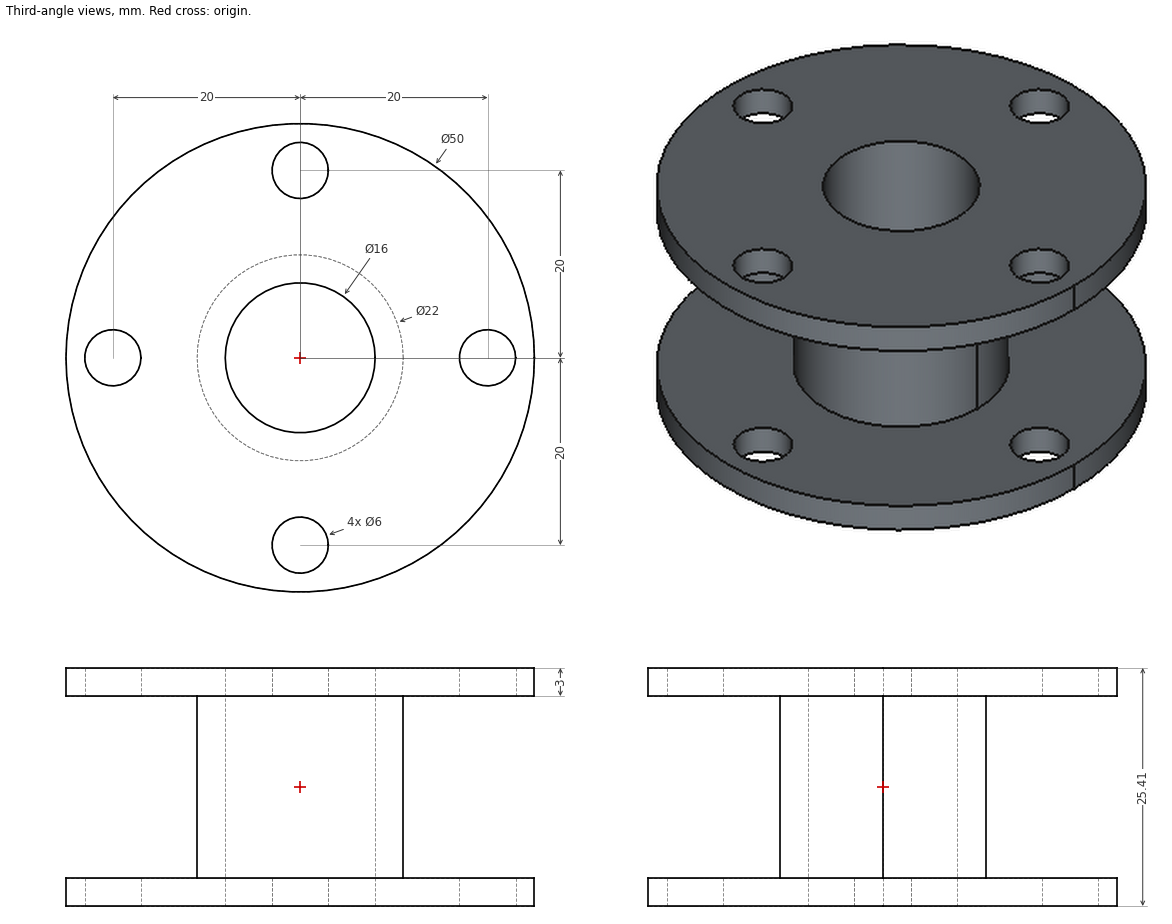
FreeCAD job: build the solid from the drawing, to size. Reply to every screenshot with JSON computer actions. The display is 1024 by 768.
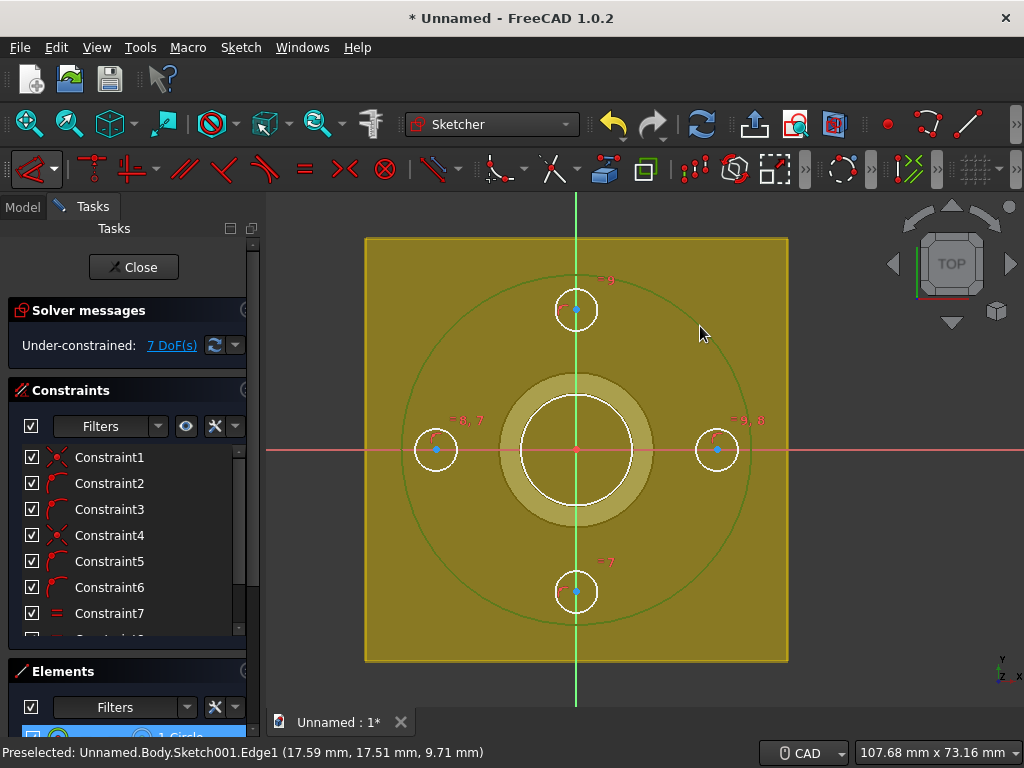
{"action": "left_click", "coordinate": [56, 170]}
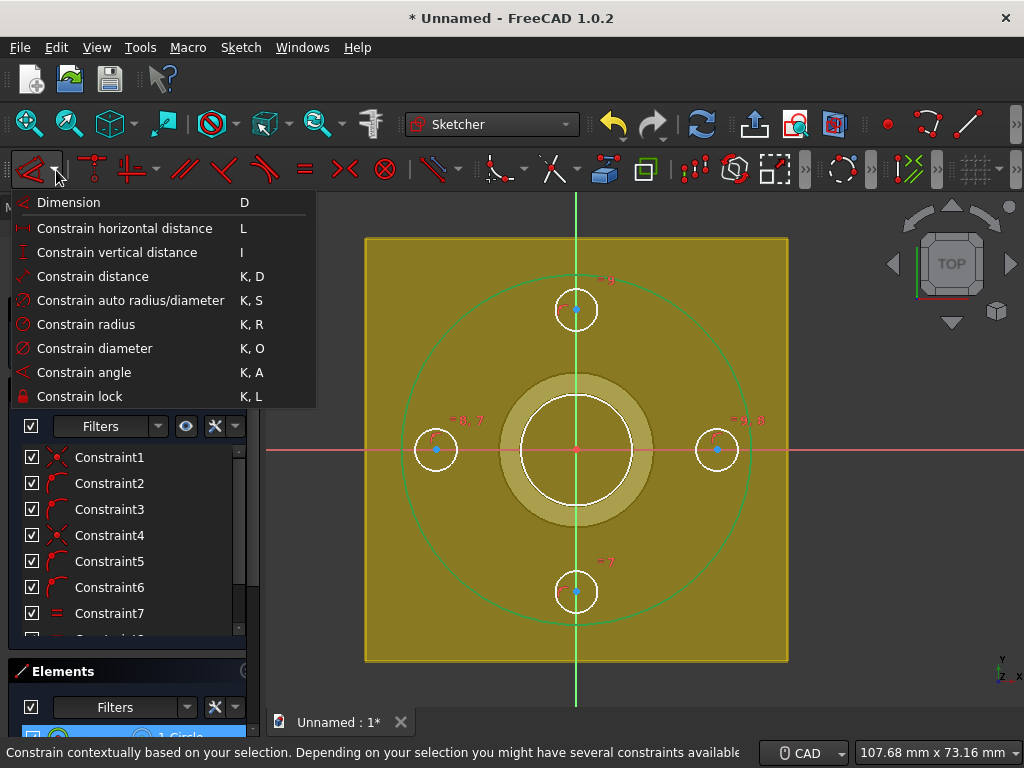
{"action": "left_click", "coordinate": [164, 348]}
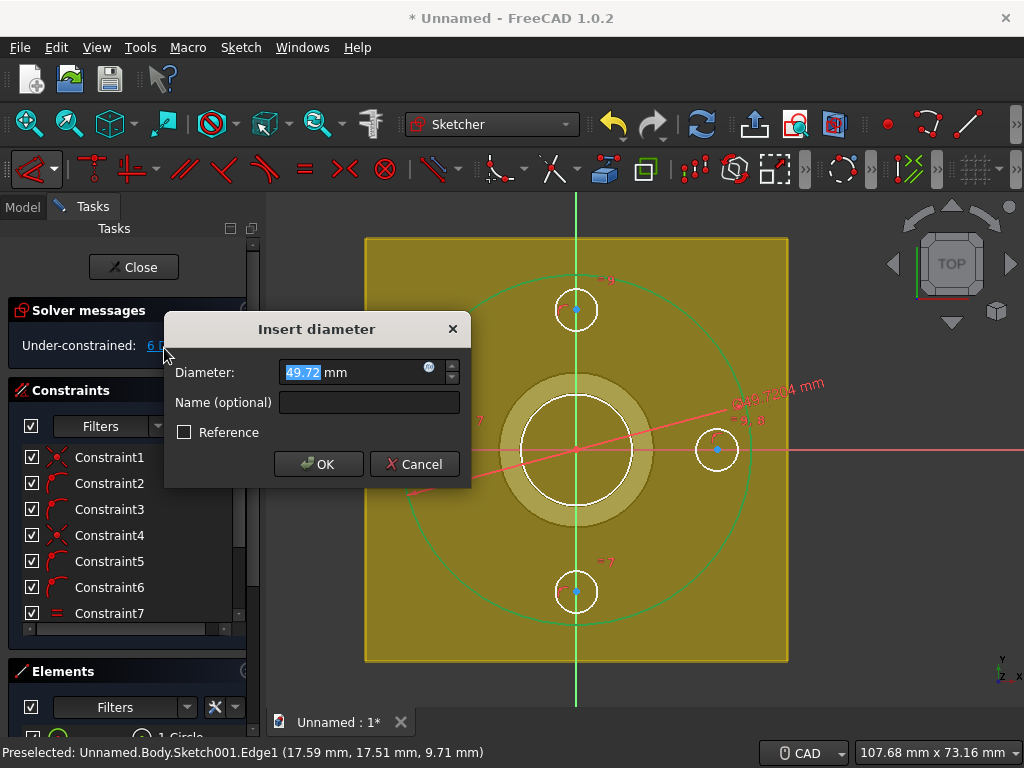
{"action": "type", "text": "50"}
{"action": "key", "text": "Return"}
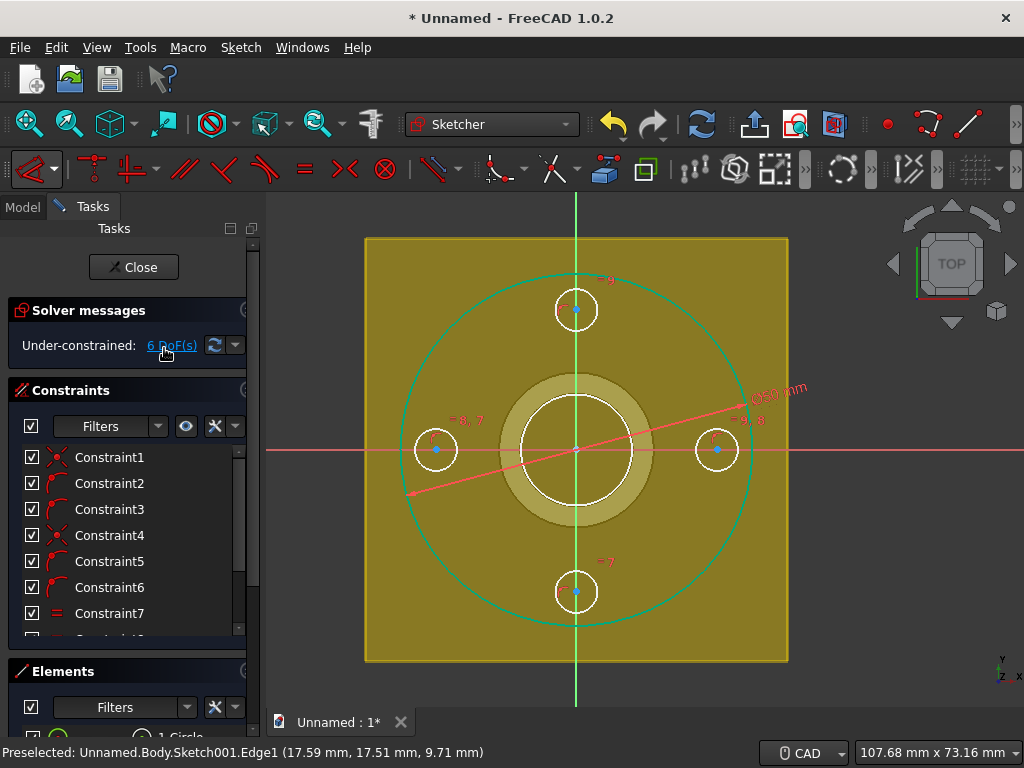
{"action": "left_click", "coordinate": [591, 577]}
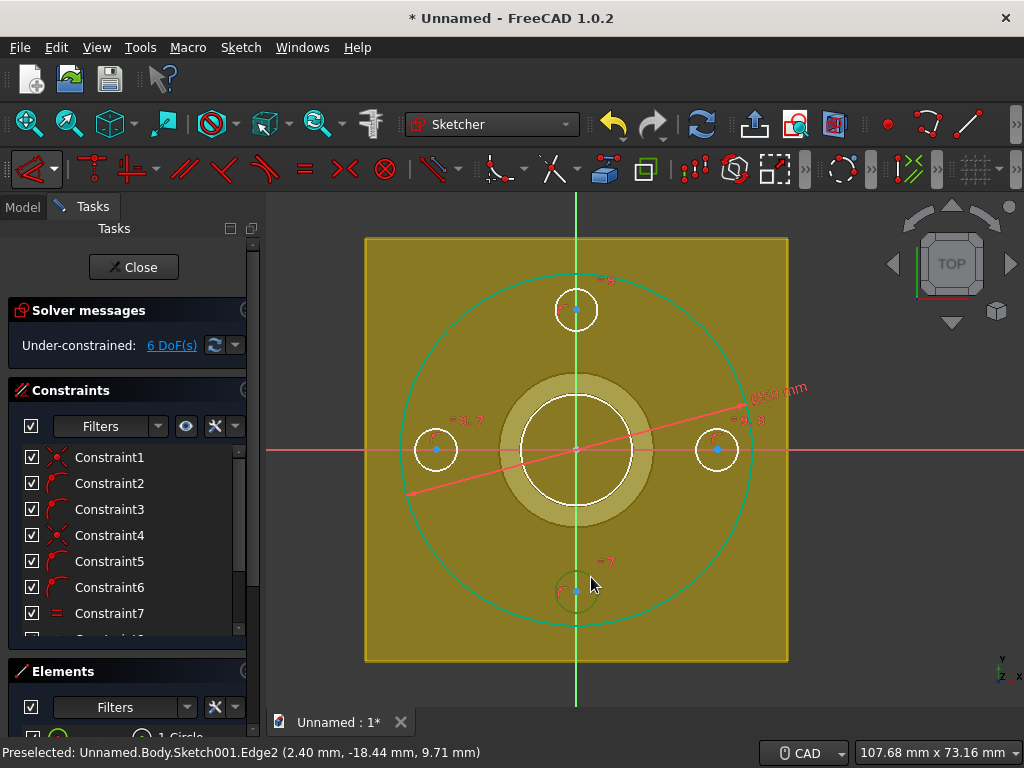
{"action": "key", "text": "k o"}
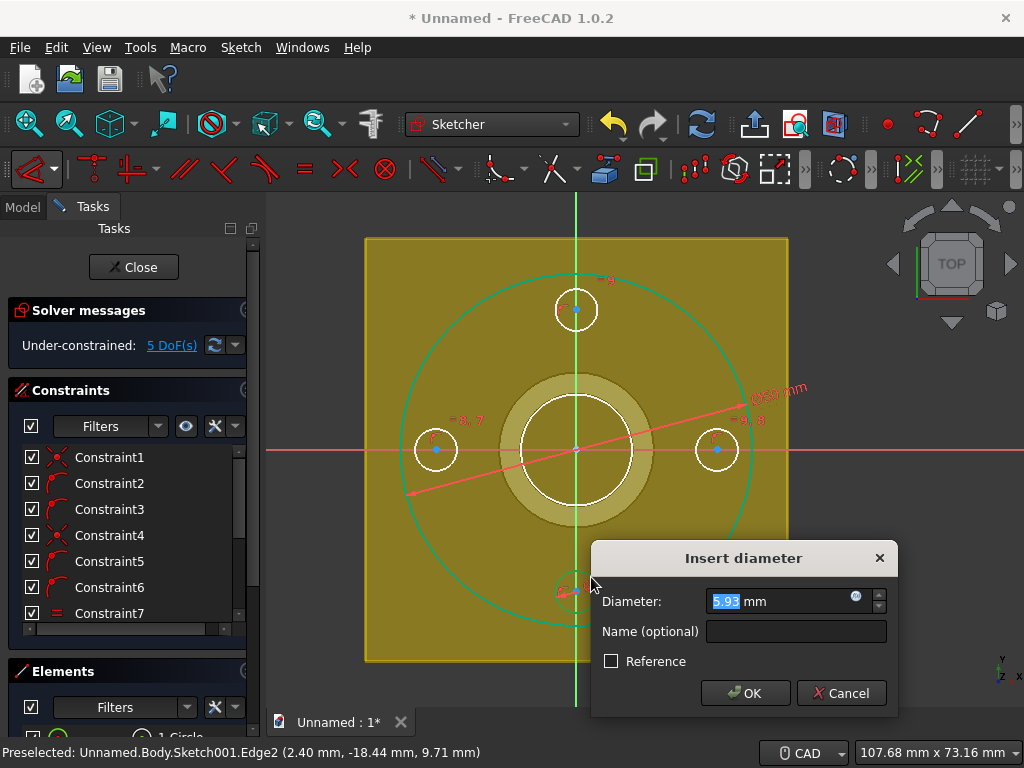
{"action": "type", "text": "6"}
{"action": "key", "text": "Return"}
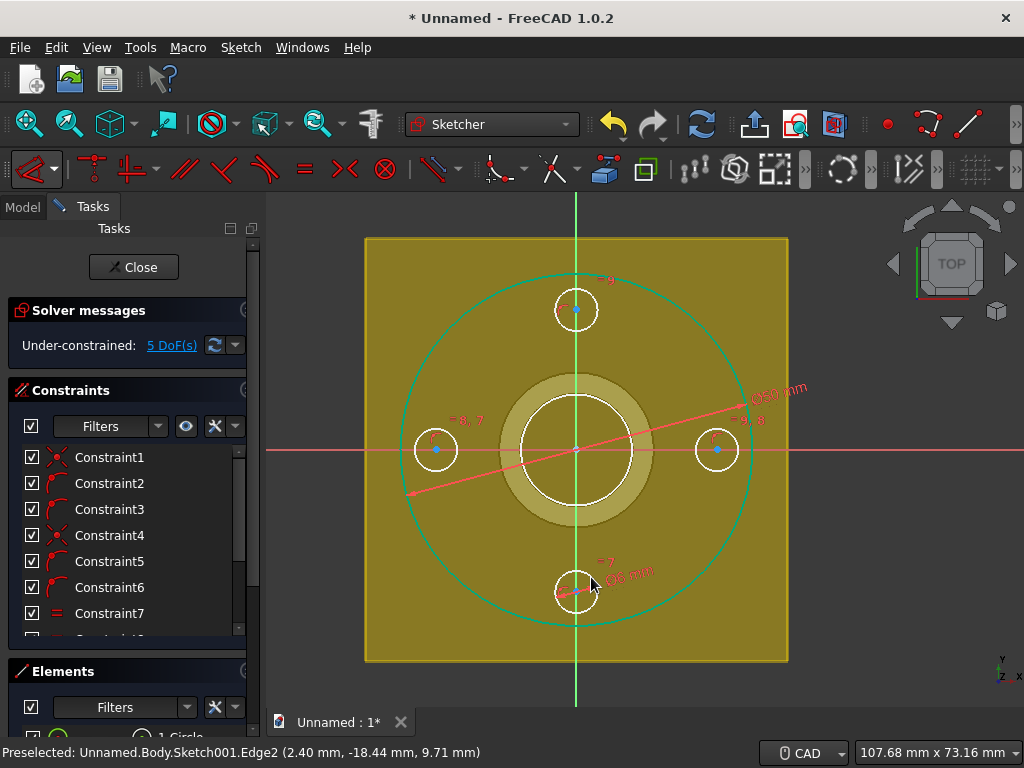
{"action": "left_click", "coordinate": [616, 411]}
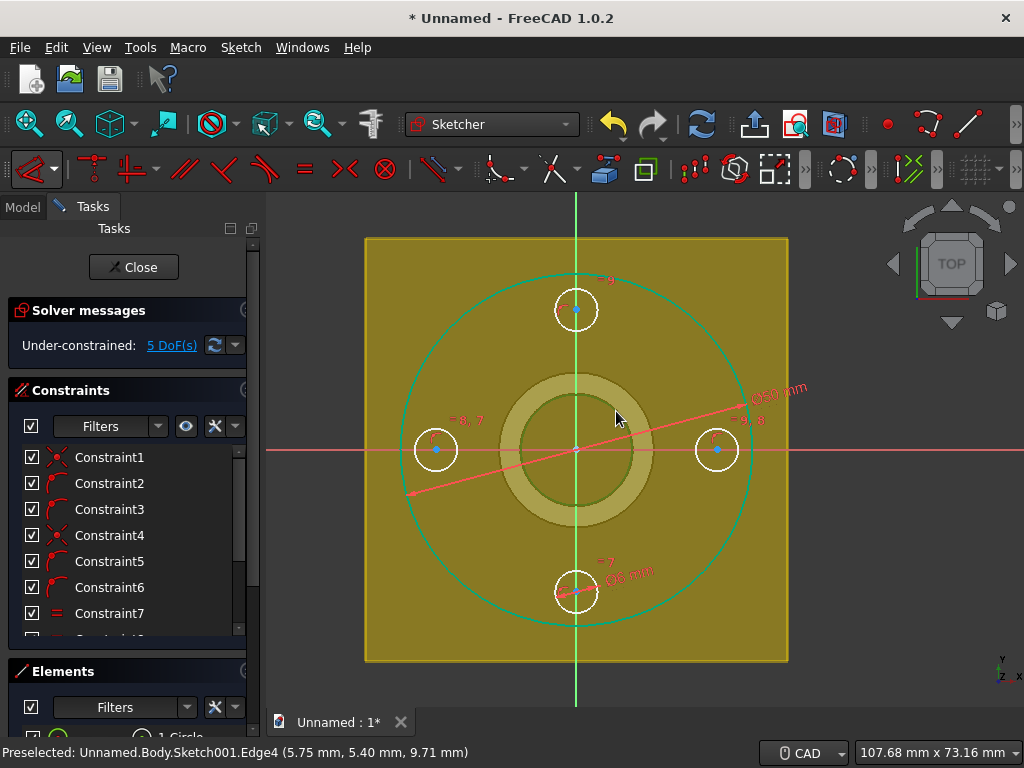
{"action": "left_click", "coordinate": [56, 170]}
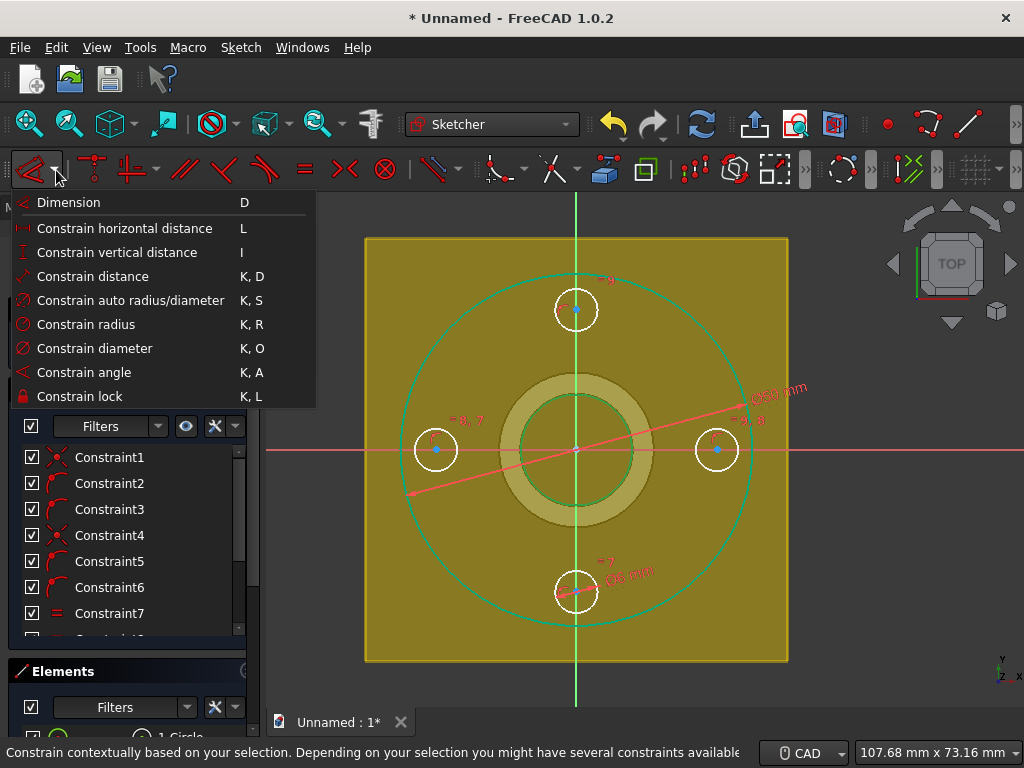
{"action": "left_click", "coordinate": [164, 348]}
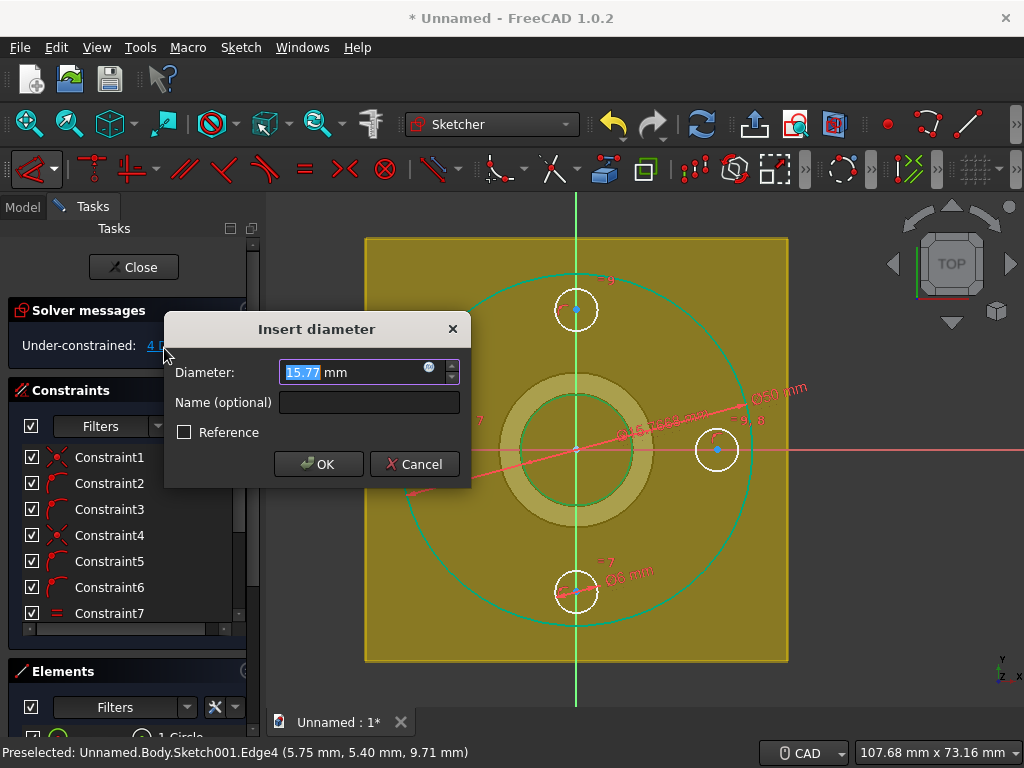
{"action": "type", "text": "16"}
{"action": "key", "text": "Return"}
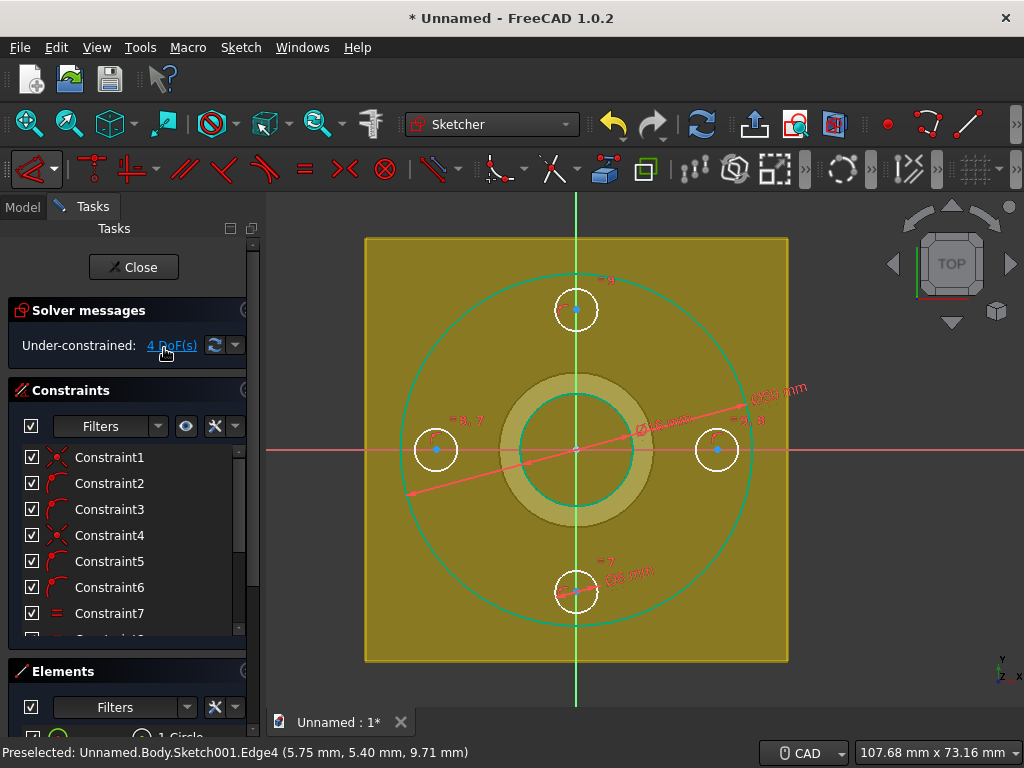
{"action": "left_click", "coordinate": [576, 592]}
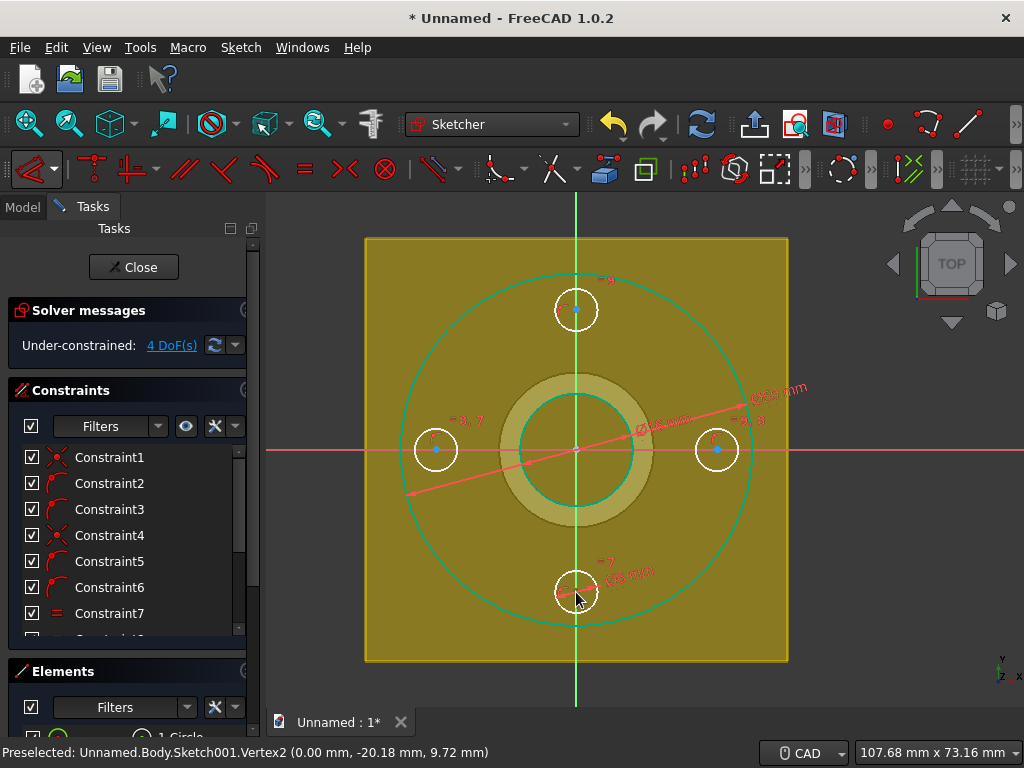
{"action": "left_click", "coordinate": [56, 170]}